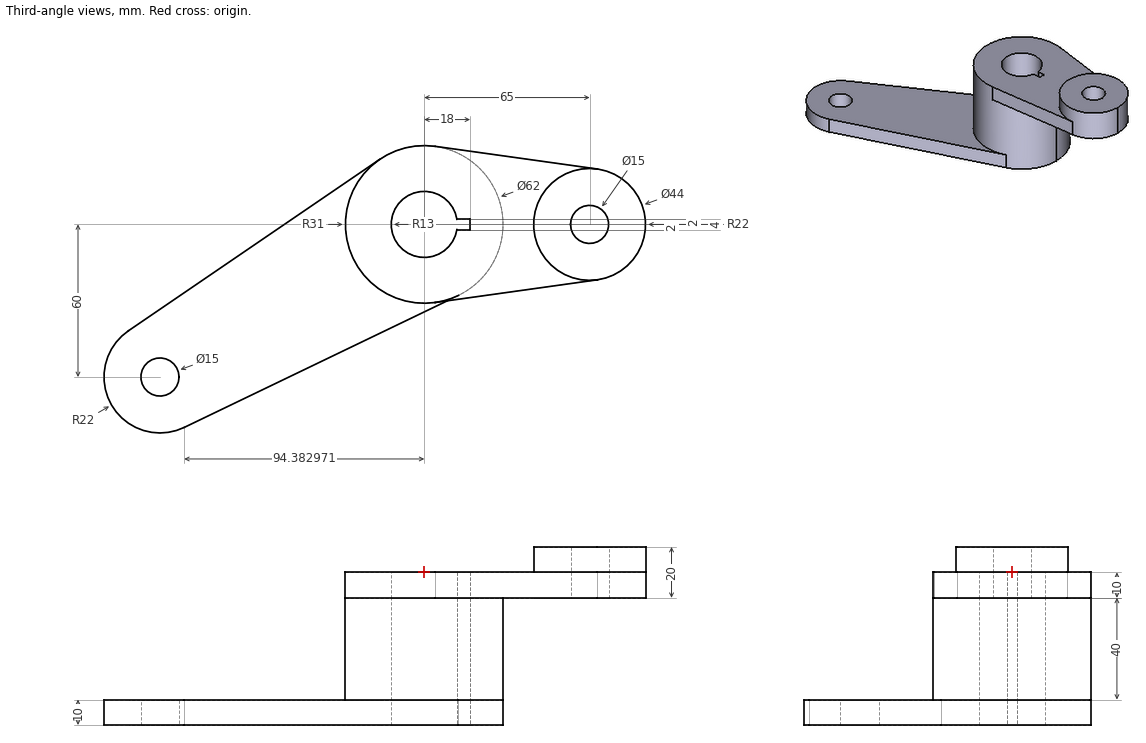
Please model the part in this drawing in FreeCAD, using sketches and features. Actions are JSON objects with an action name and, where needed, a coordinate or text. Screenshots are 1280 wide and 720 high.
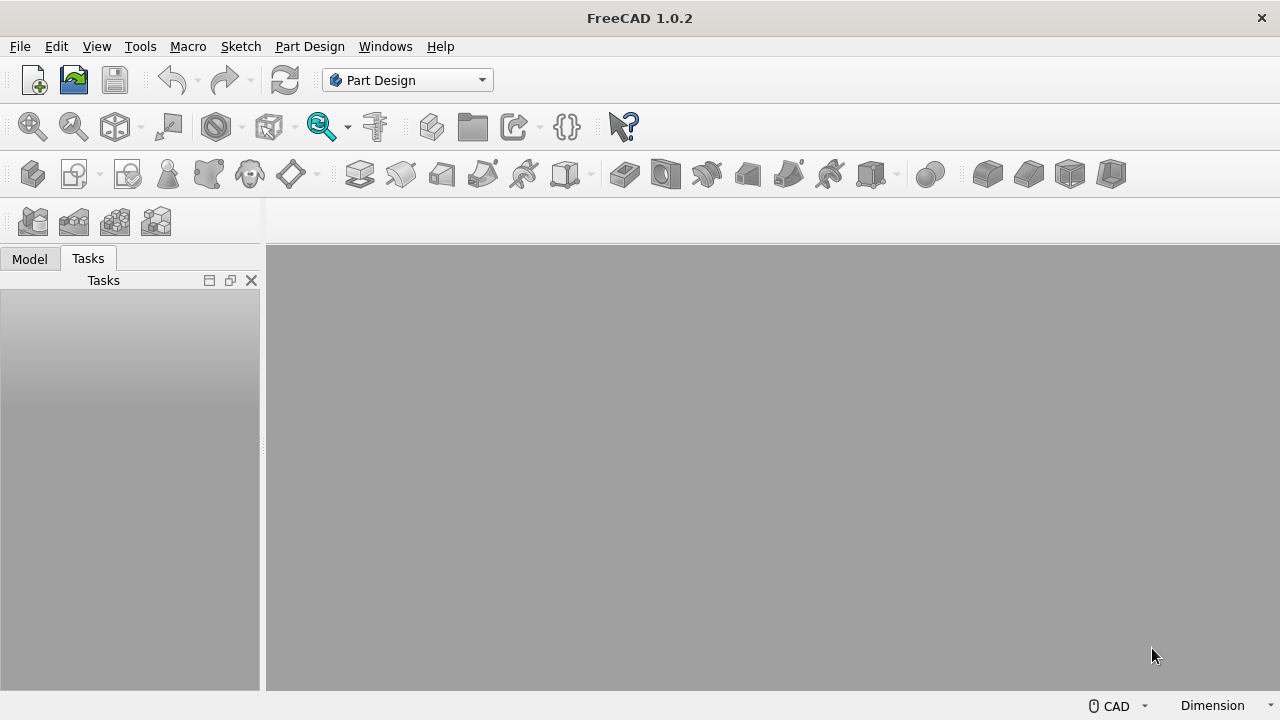
{"action": "key", "text": "ctrl+n"}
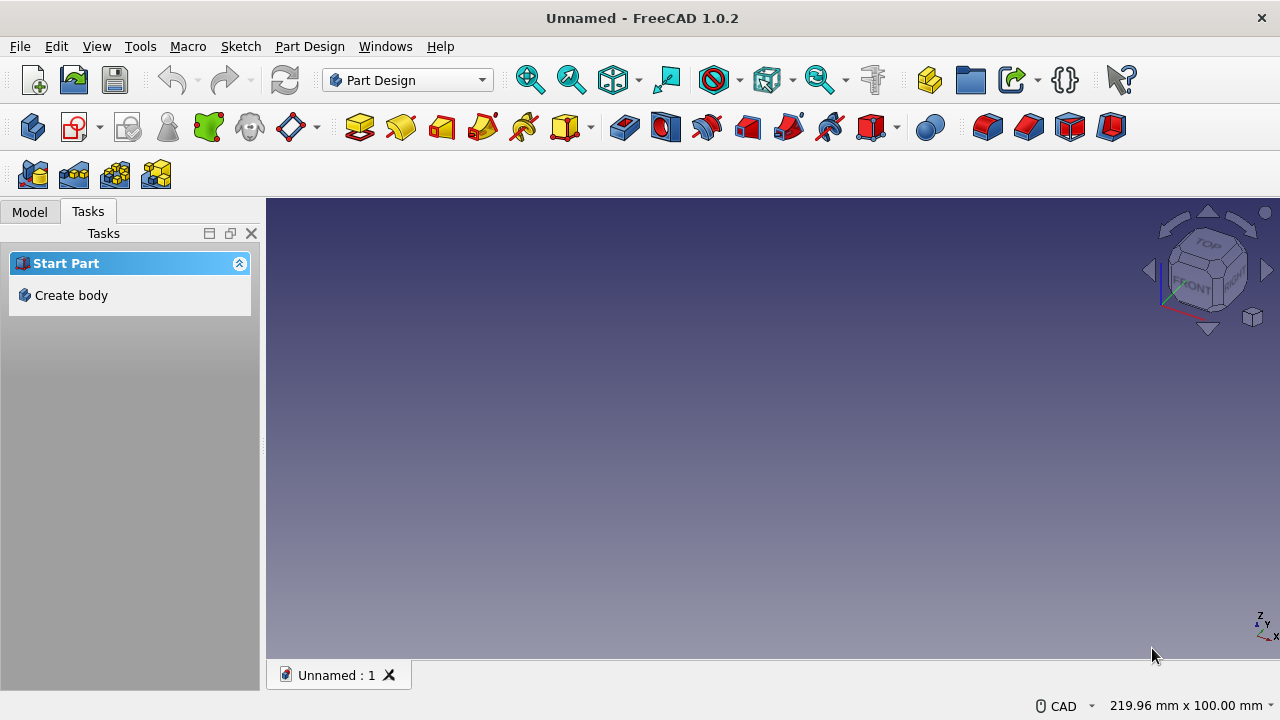
{"action": "left_click", "coordinate": [74, 128]}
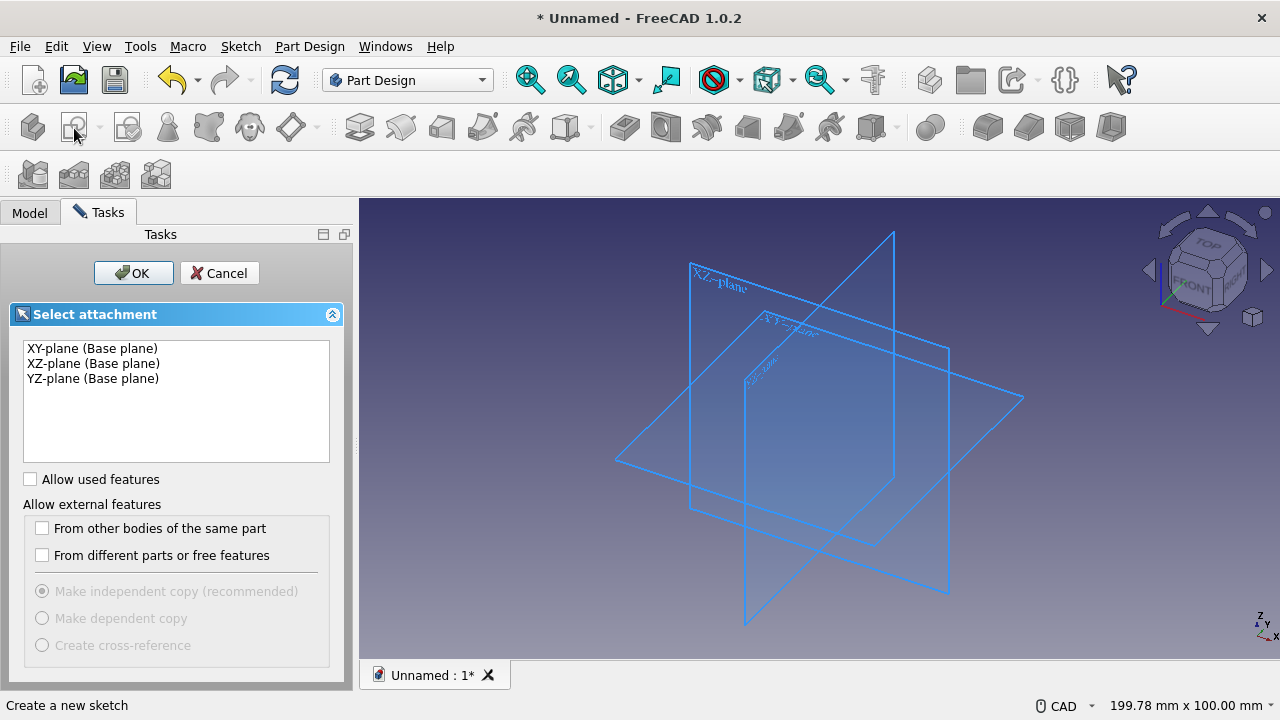
{"action": "left_click", "coordinate": [84, 348]}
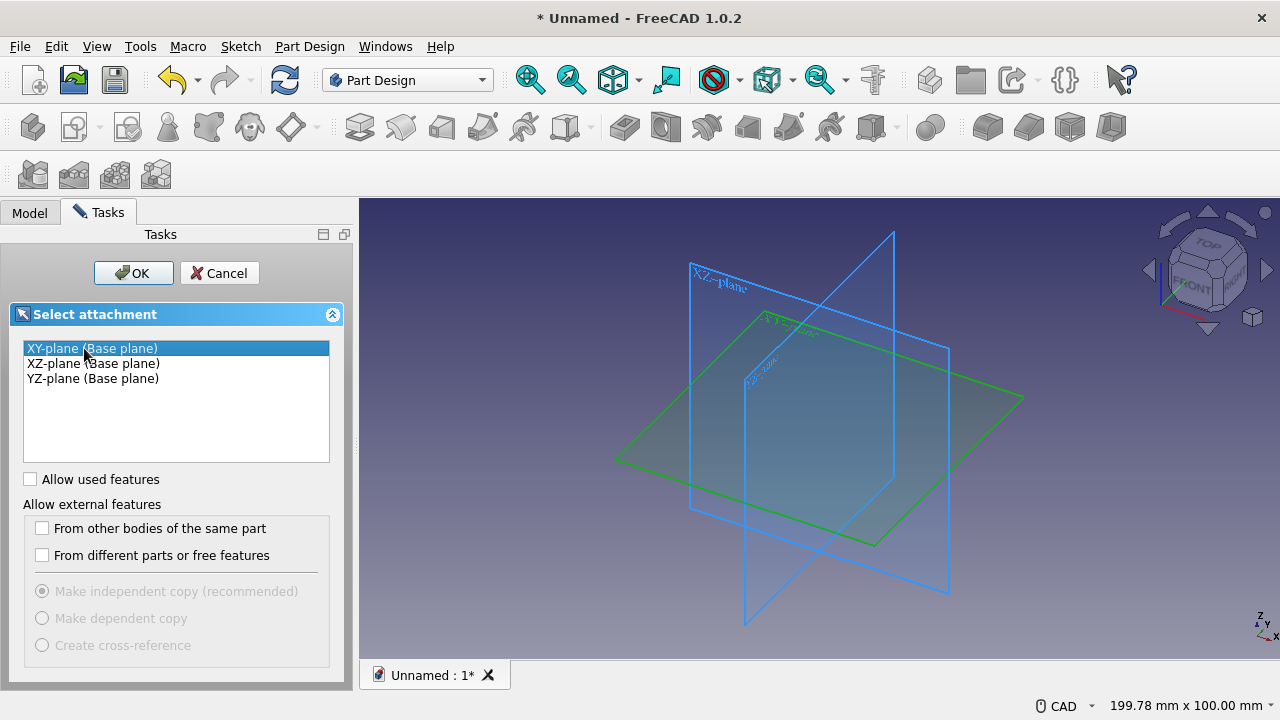
{"action": "left_click", "coordinate": [134, 273]}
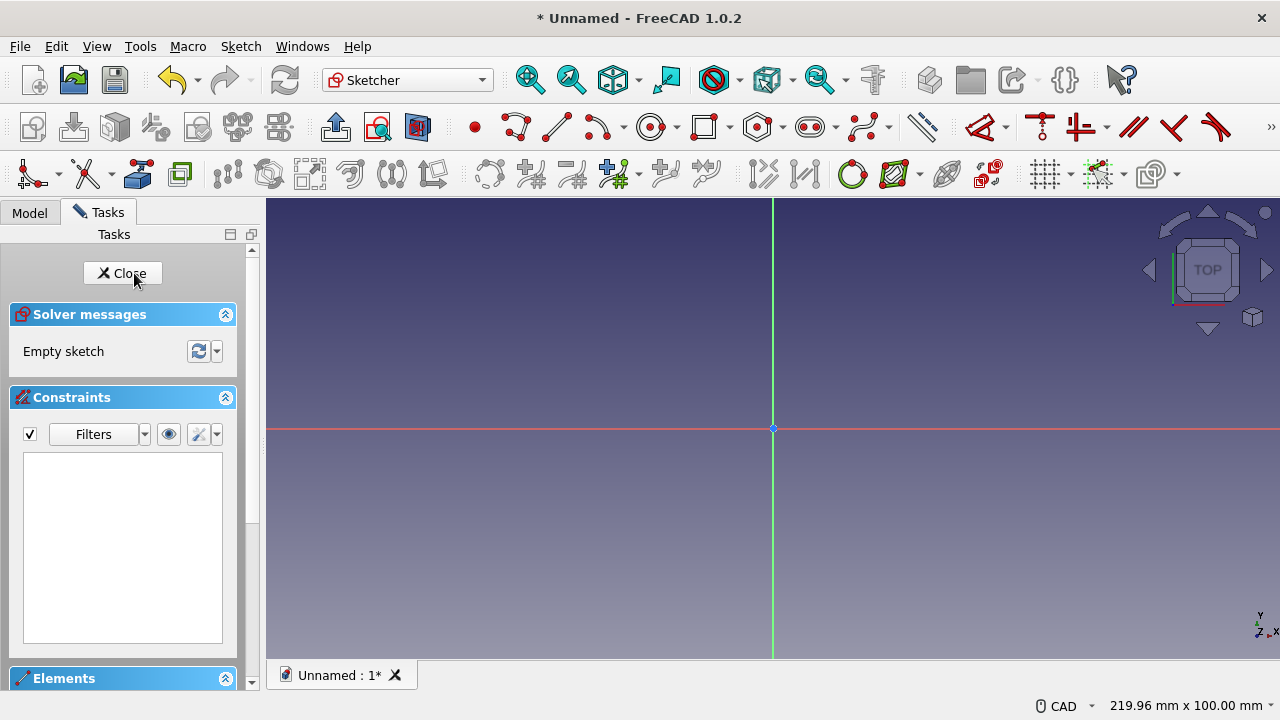
{"action": "scroll", "coordinate": [294, 428], "scroll_direction": "down", "scroll_amount": 1}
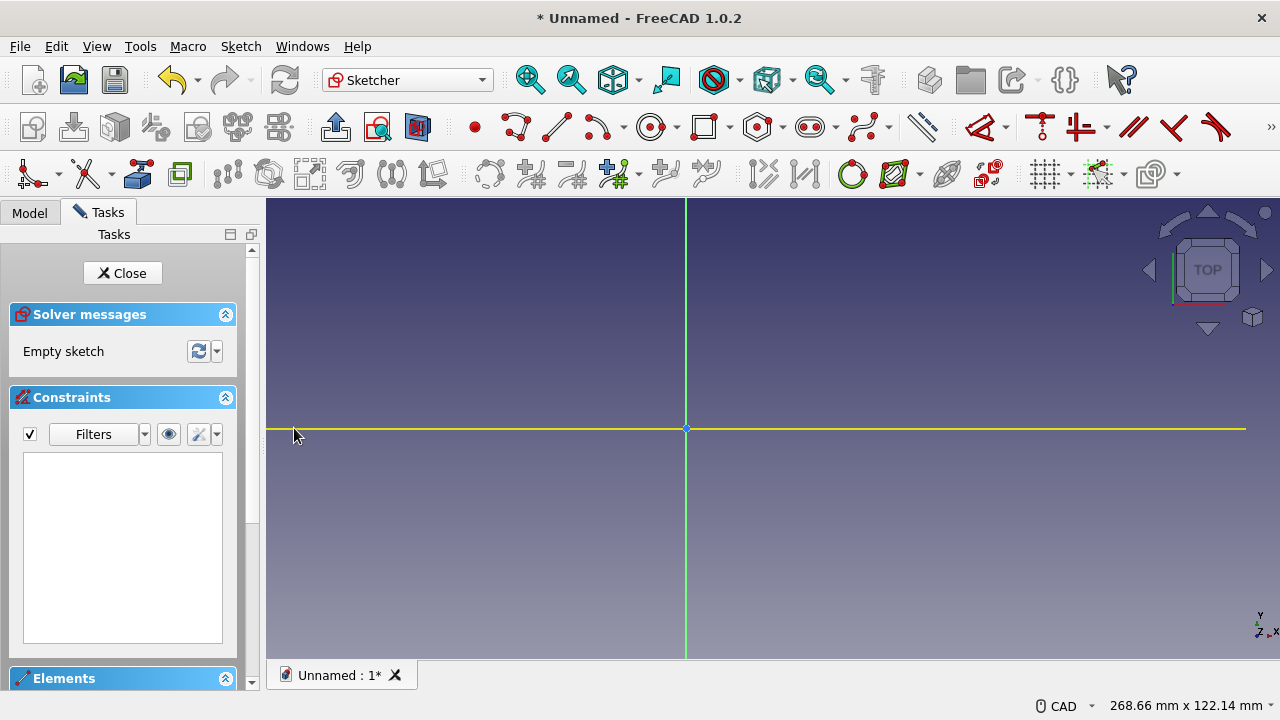
{"action": "key", "text": "g l"}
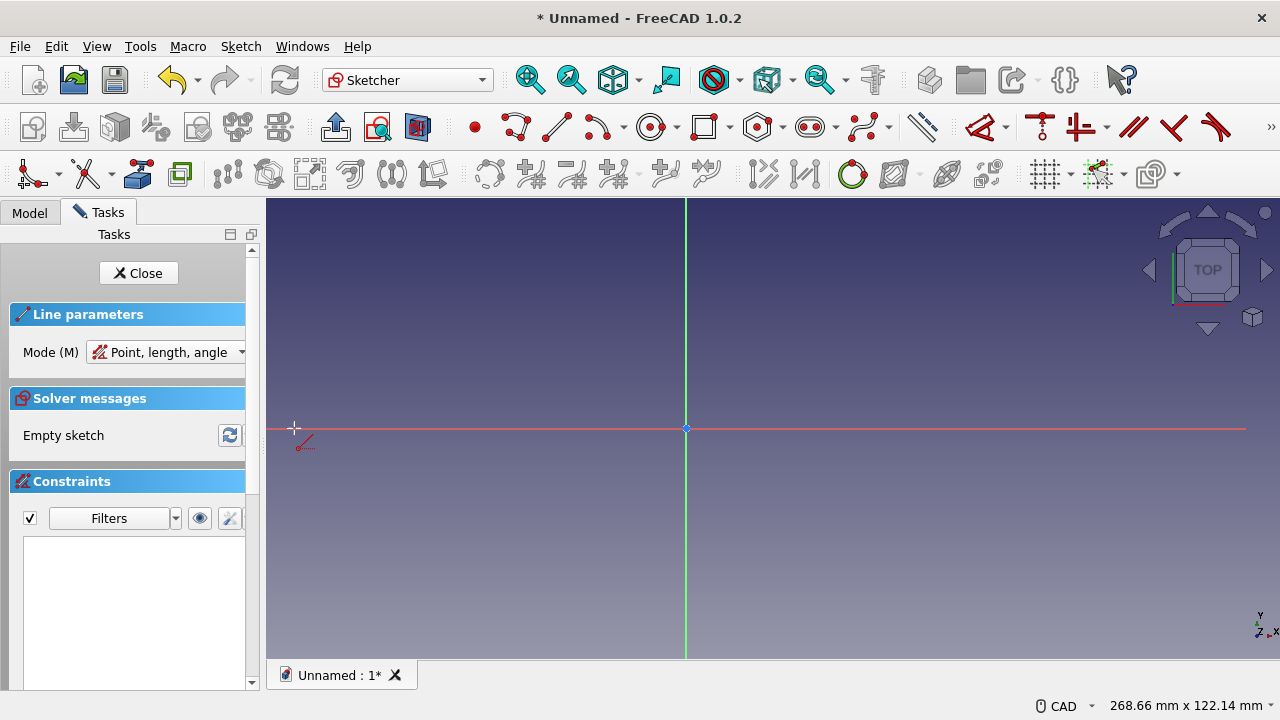
{"action": "left_click", "coordinate": [943, 346]}
{"action": "left_click", "coordinate": [702, 313]}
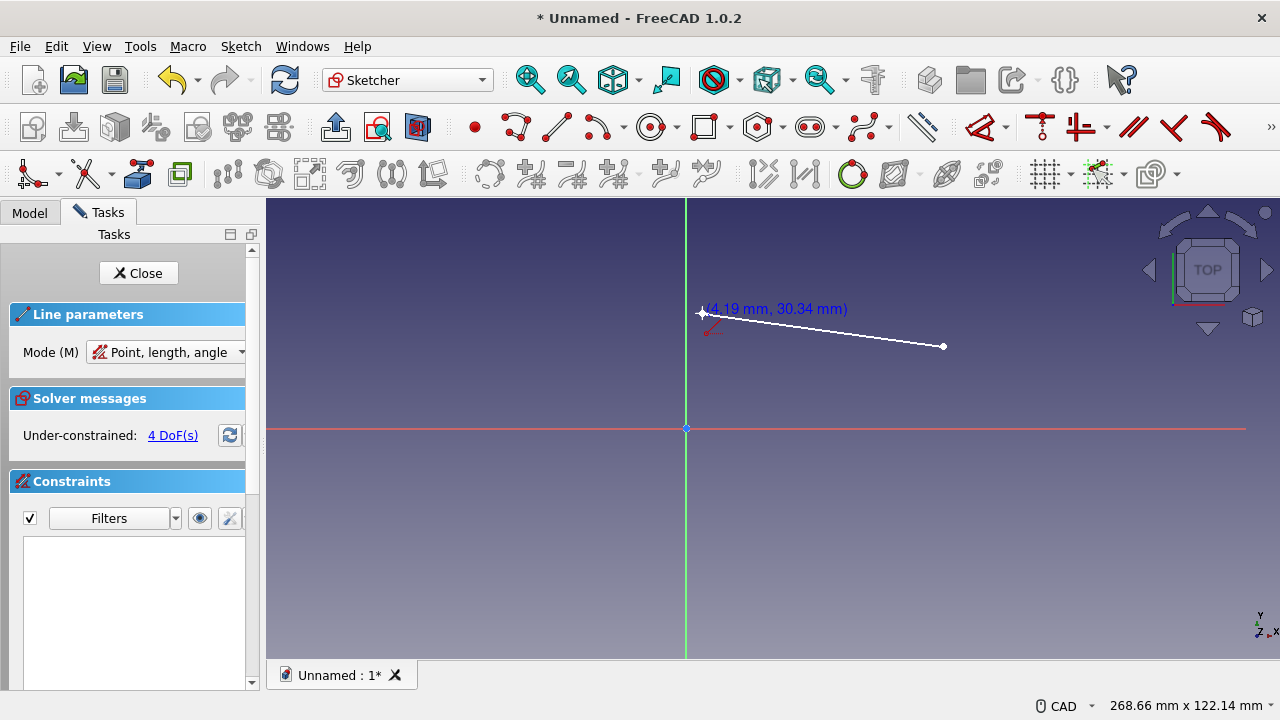
{"action": "left_click", "coordinate": [702, 544]}
{"action": "left_click", "coordinate": [943, 511]}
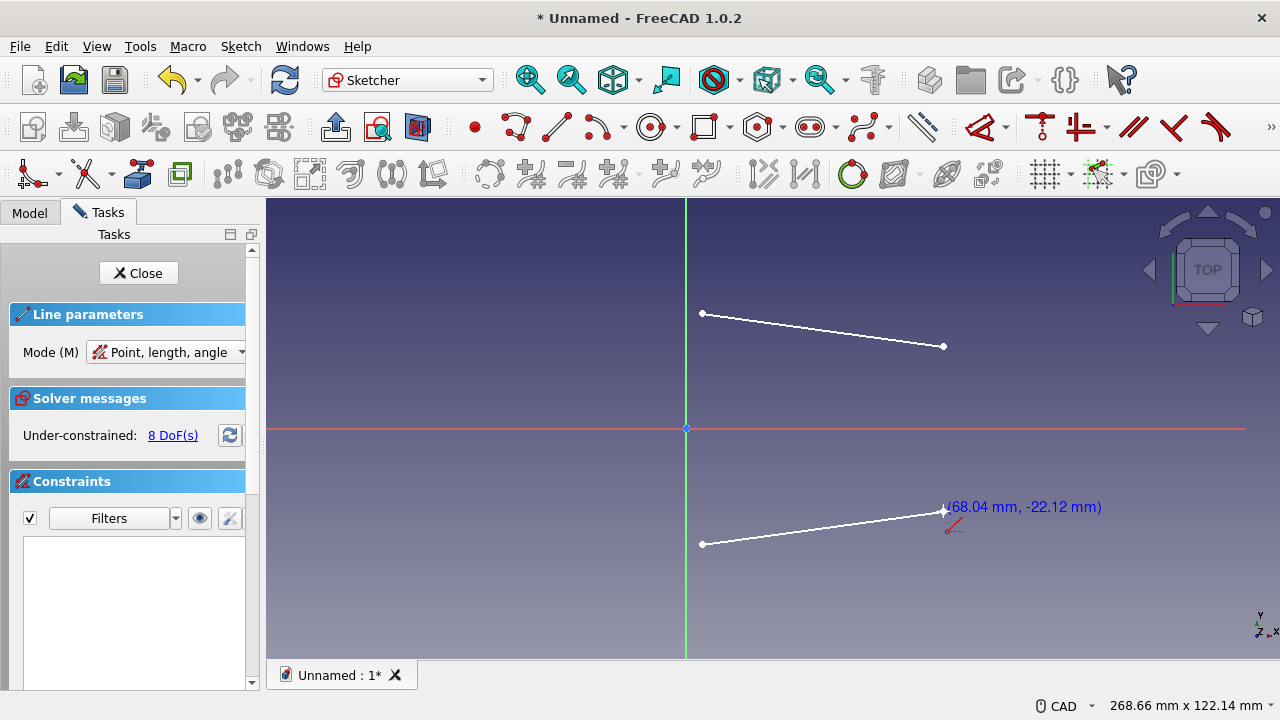
{"action": "key", "text": "g 3 a"}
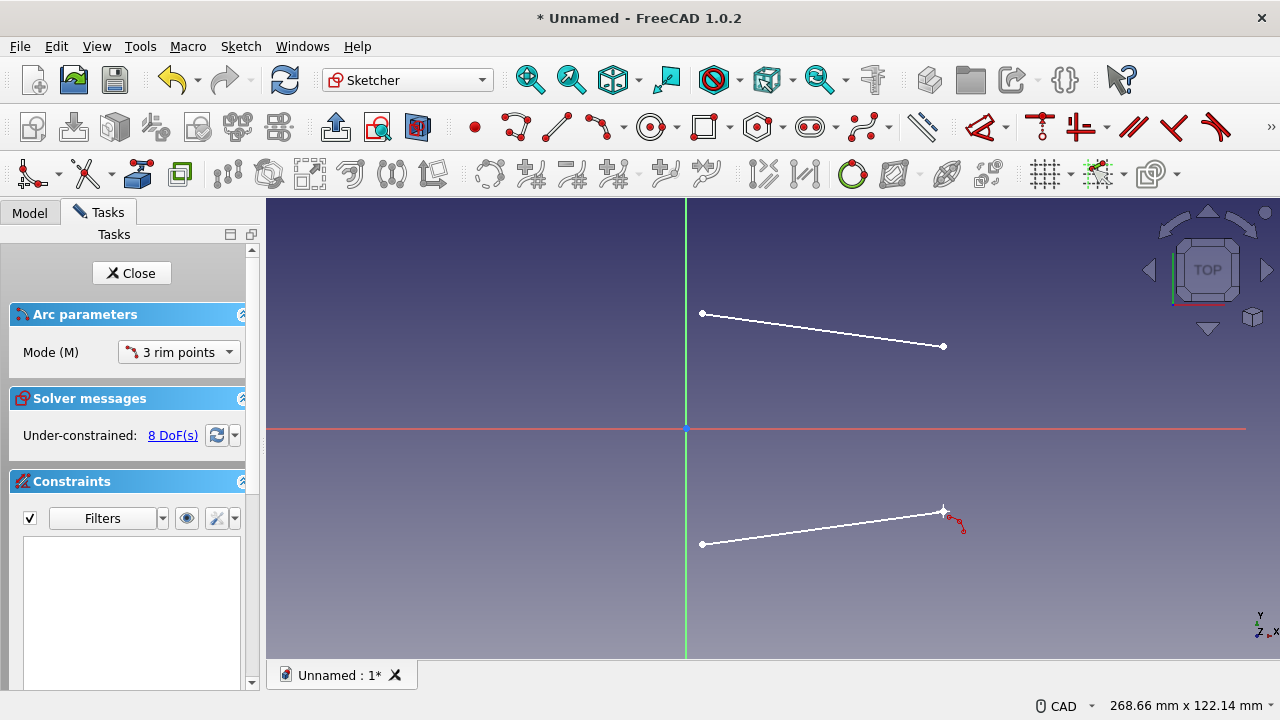
{"action": "left_click", "coordinate": [702, 314]}
{"action": "left_click", "coordinate": [702, 545]}
{"action": "left_click", "coordinate": [576, 389]}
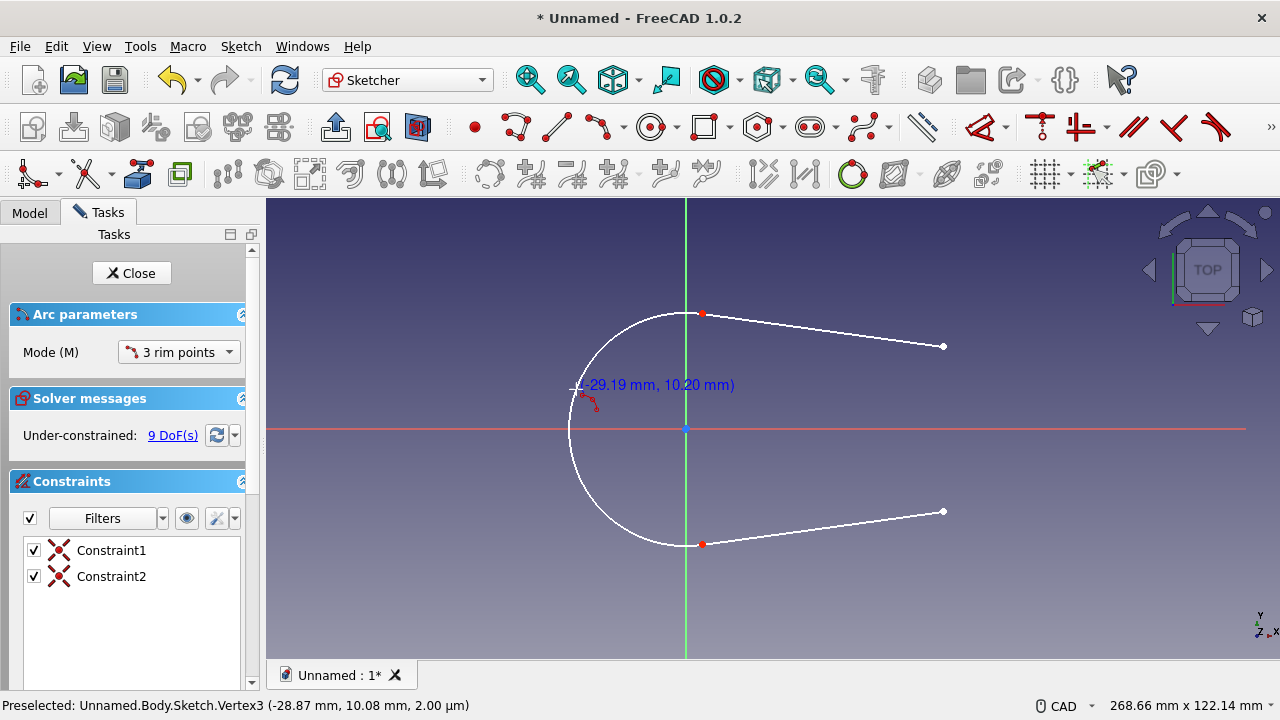
{"action": "left_click", "coordinate": [943, 512]}
{"action": "left_click", "coordinate": [943, 347]}
{"action": "left_click", "coordinate": [1011, 452]}
{"action": "key", "text": "Escape"}